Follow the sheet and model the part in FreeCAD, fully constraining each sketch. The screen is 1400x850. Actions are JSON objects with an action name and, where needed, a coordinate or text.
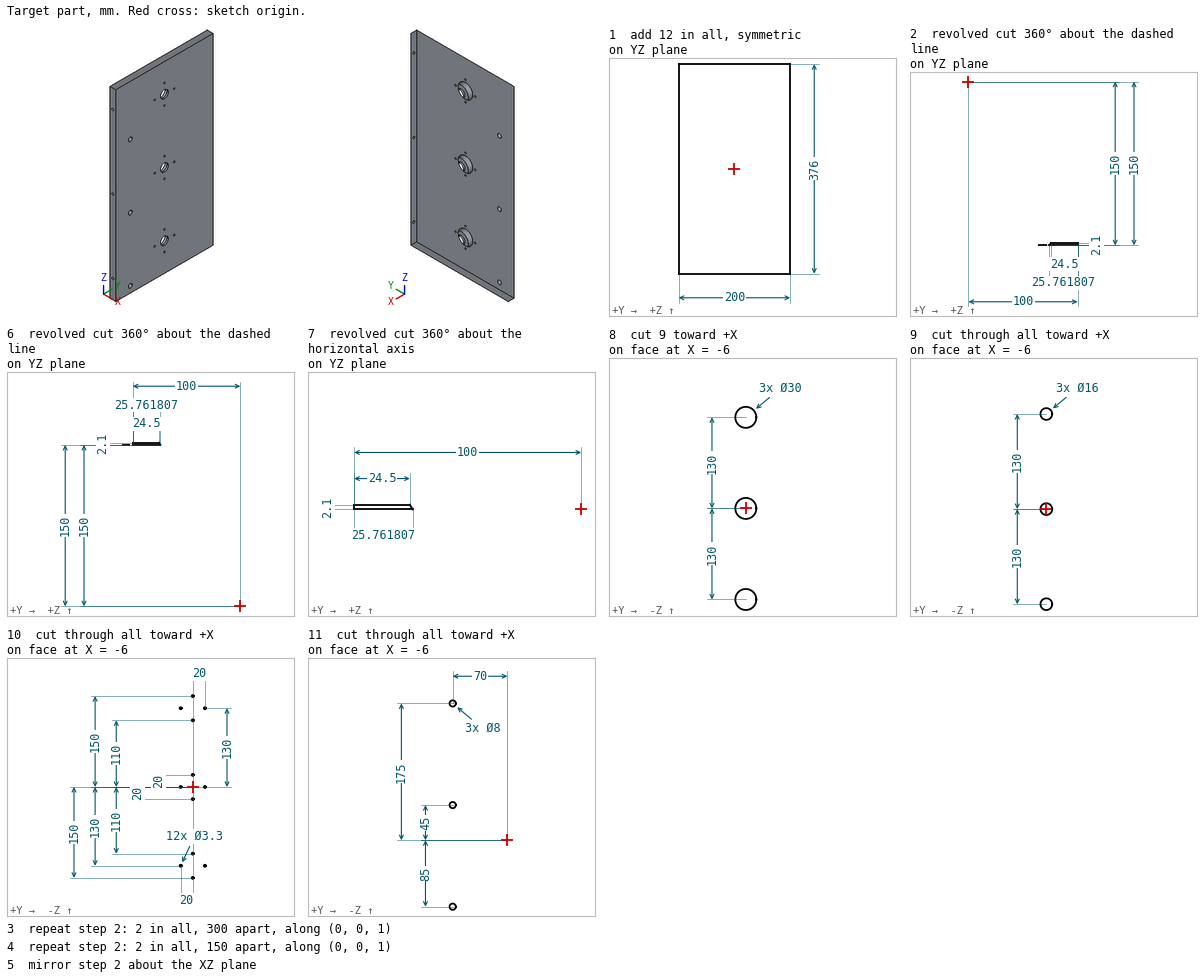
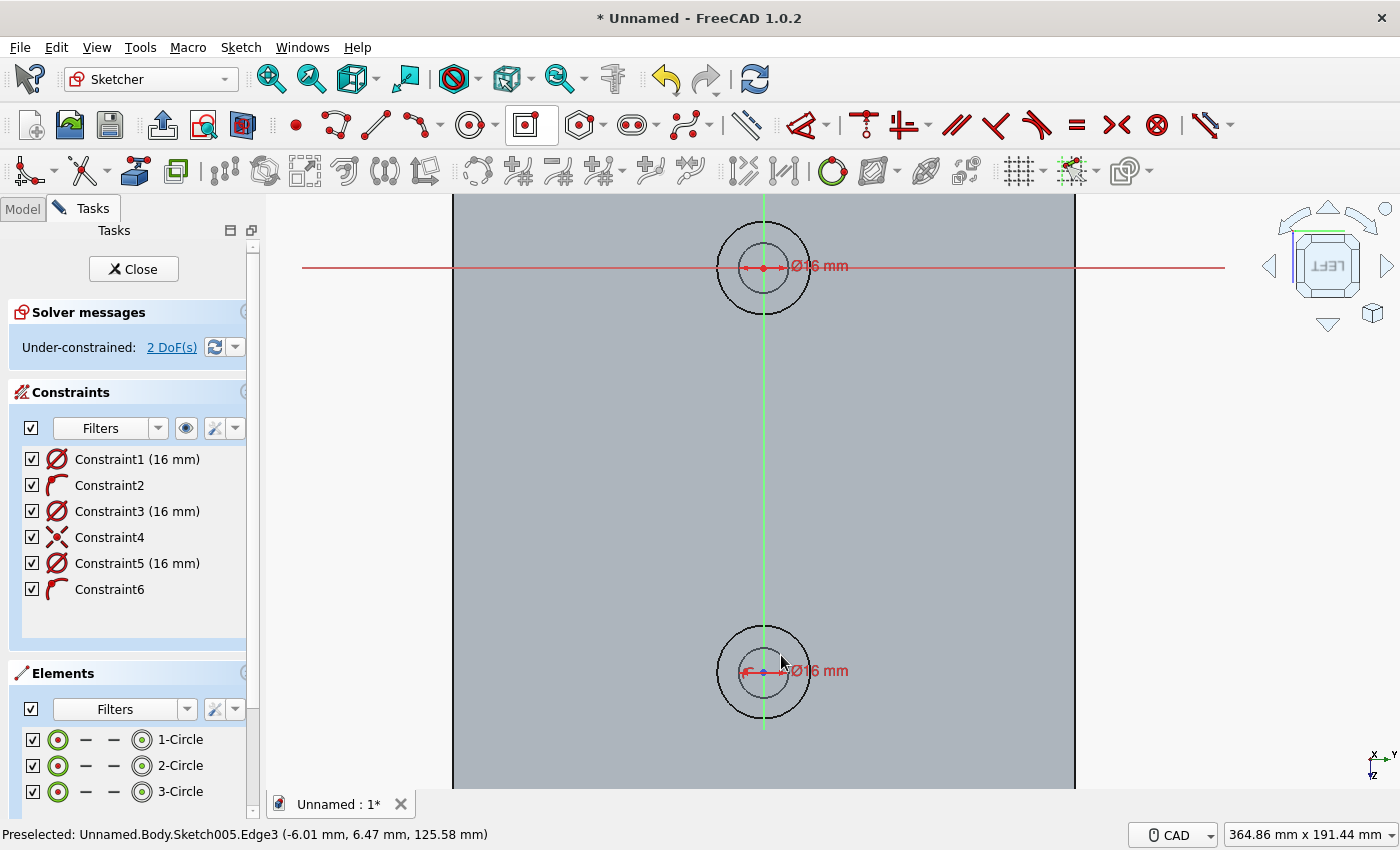
{"action": "left_click", "coordinate": [802, 126]}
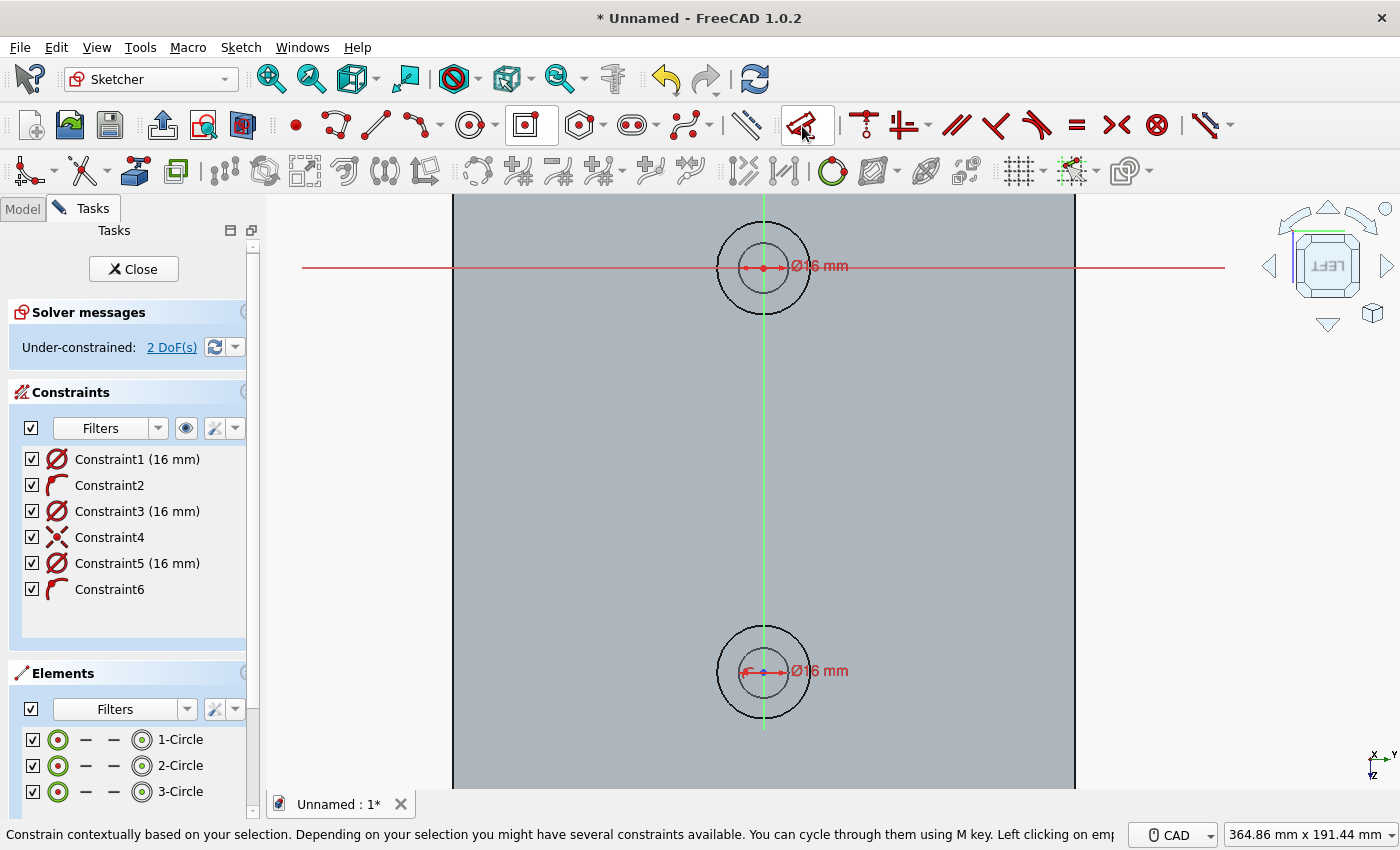
{"action": "scroll", "coordinate": [765, 674], "scroll_direction": "down", "scroll_amount": 4}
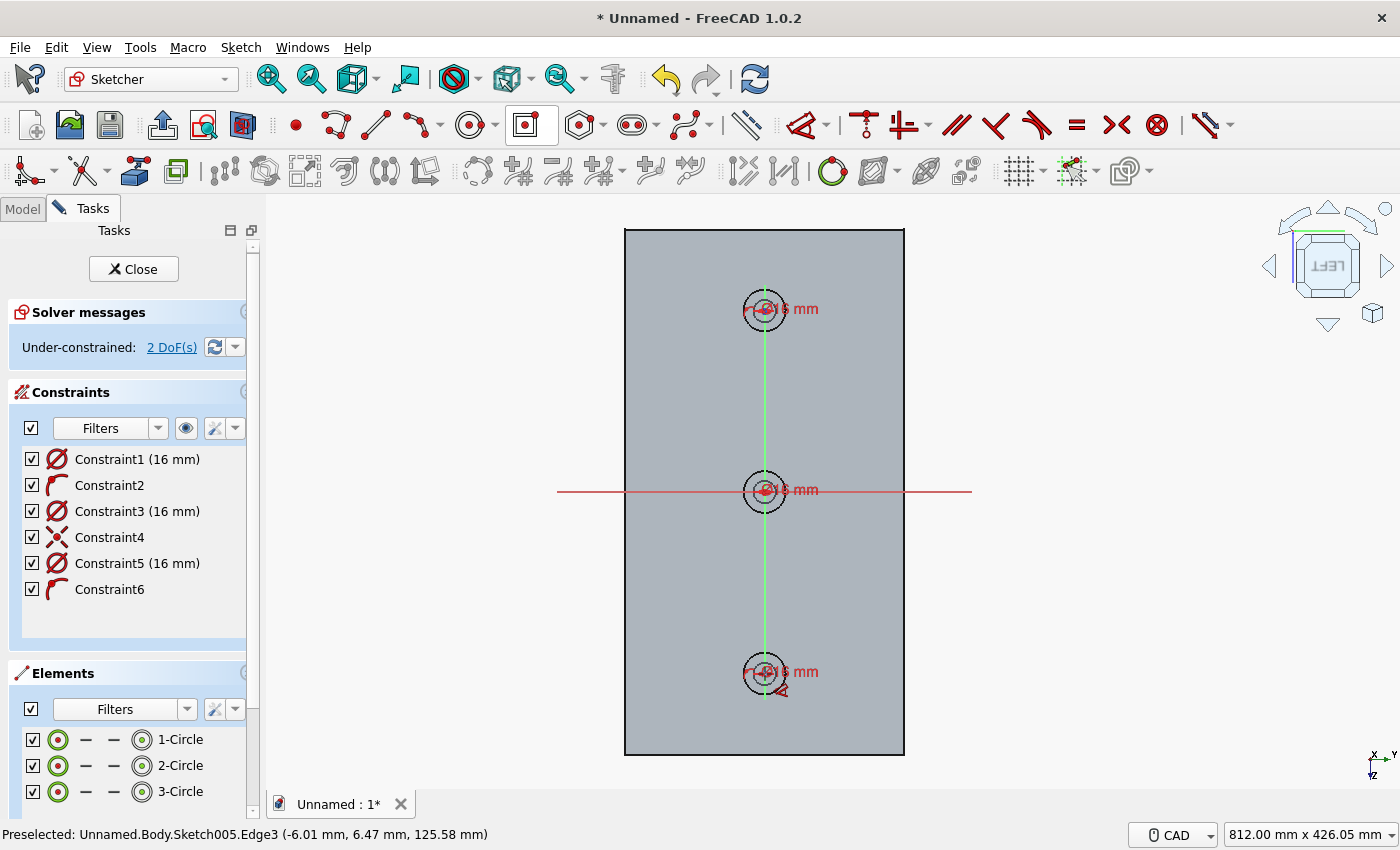
{"action": "left_click", "coordinate": [765, 311]}
{"action": "left_click", "coordinate": [799, 402]}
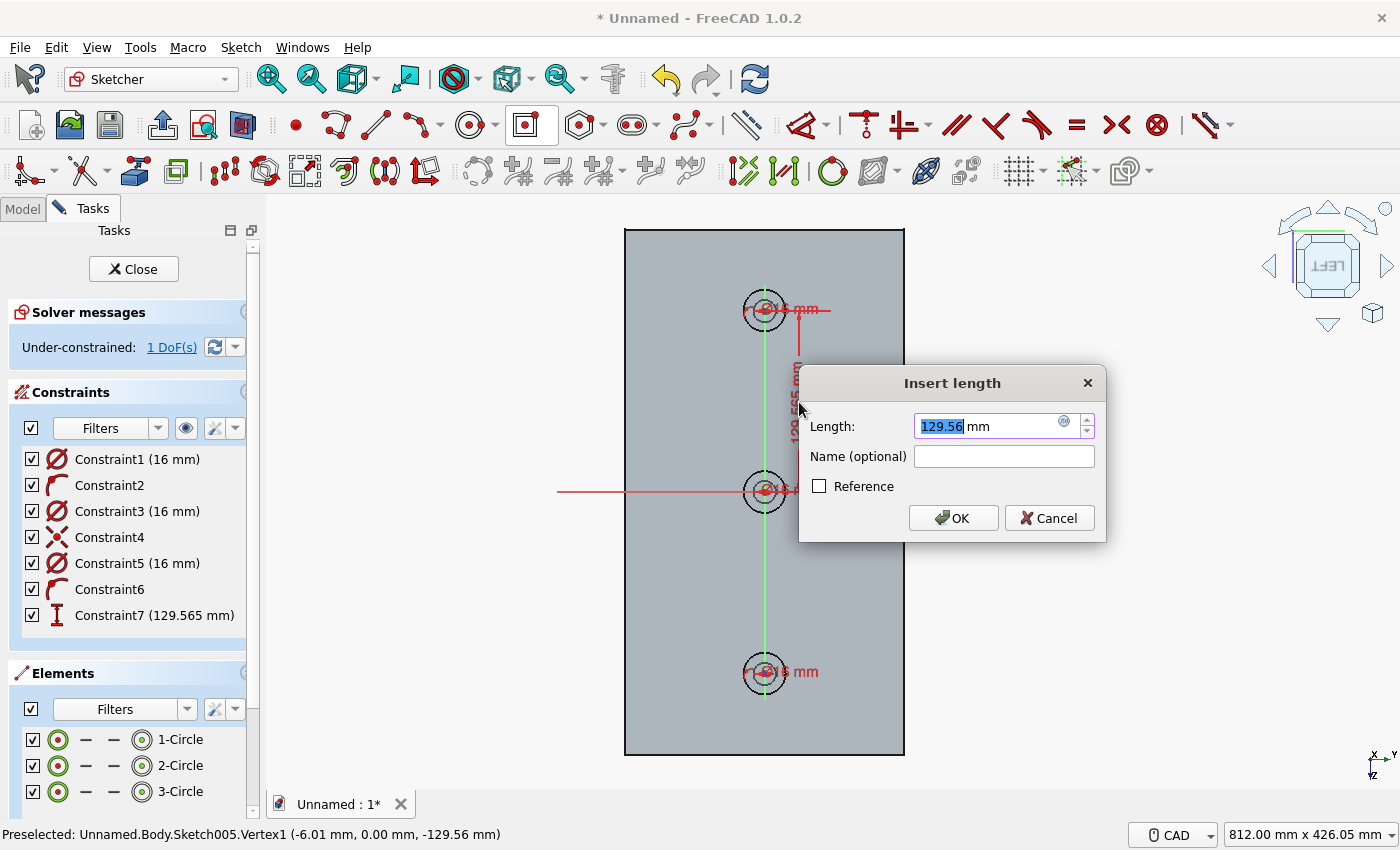
{"action": "type", "text": "130"}
{"action": "key", "text": "Return"}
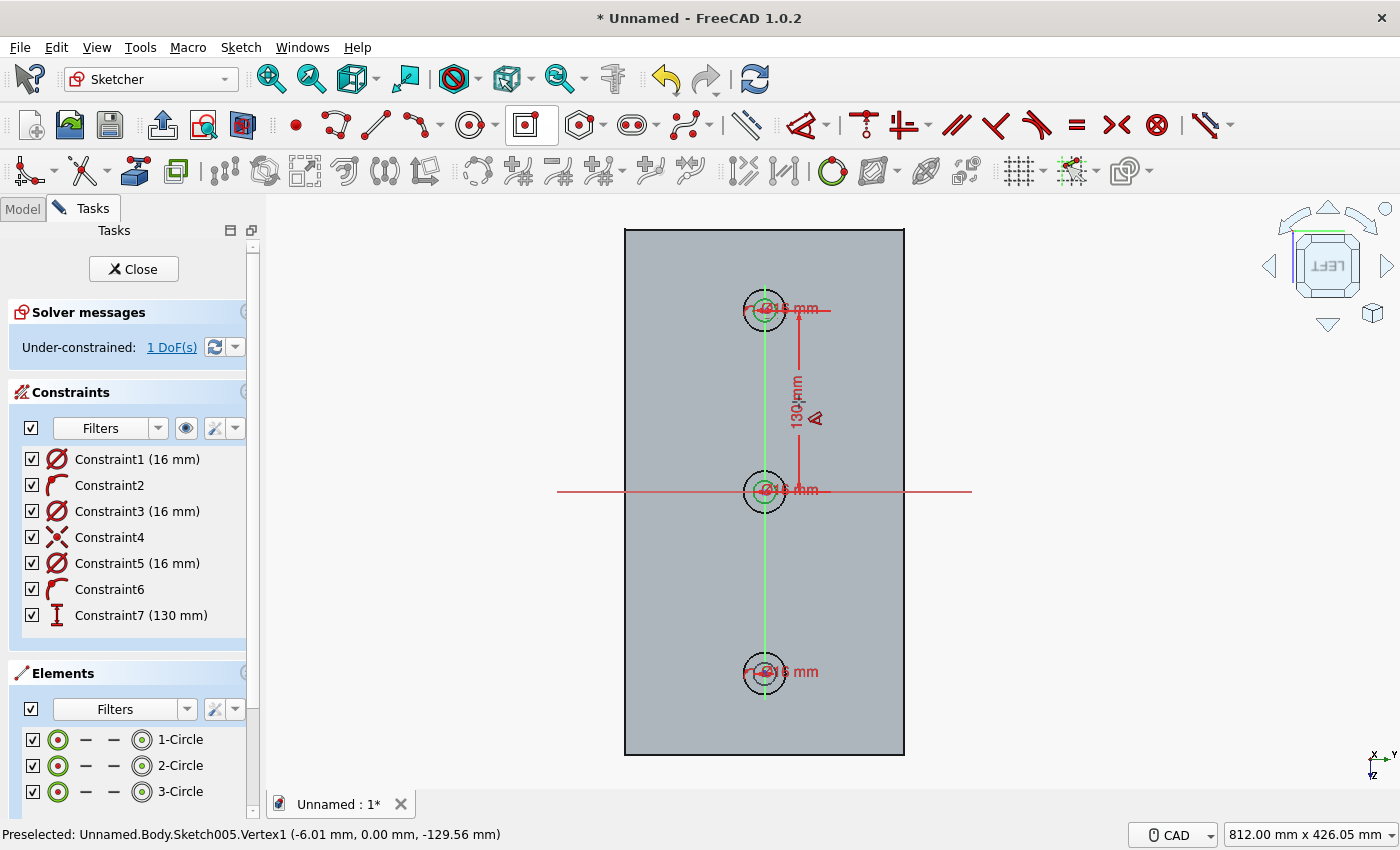
{"action": "left_click", "coordinate": [765, 674]}
{"action": "left_click", "coordinate": [799, 583]}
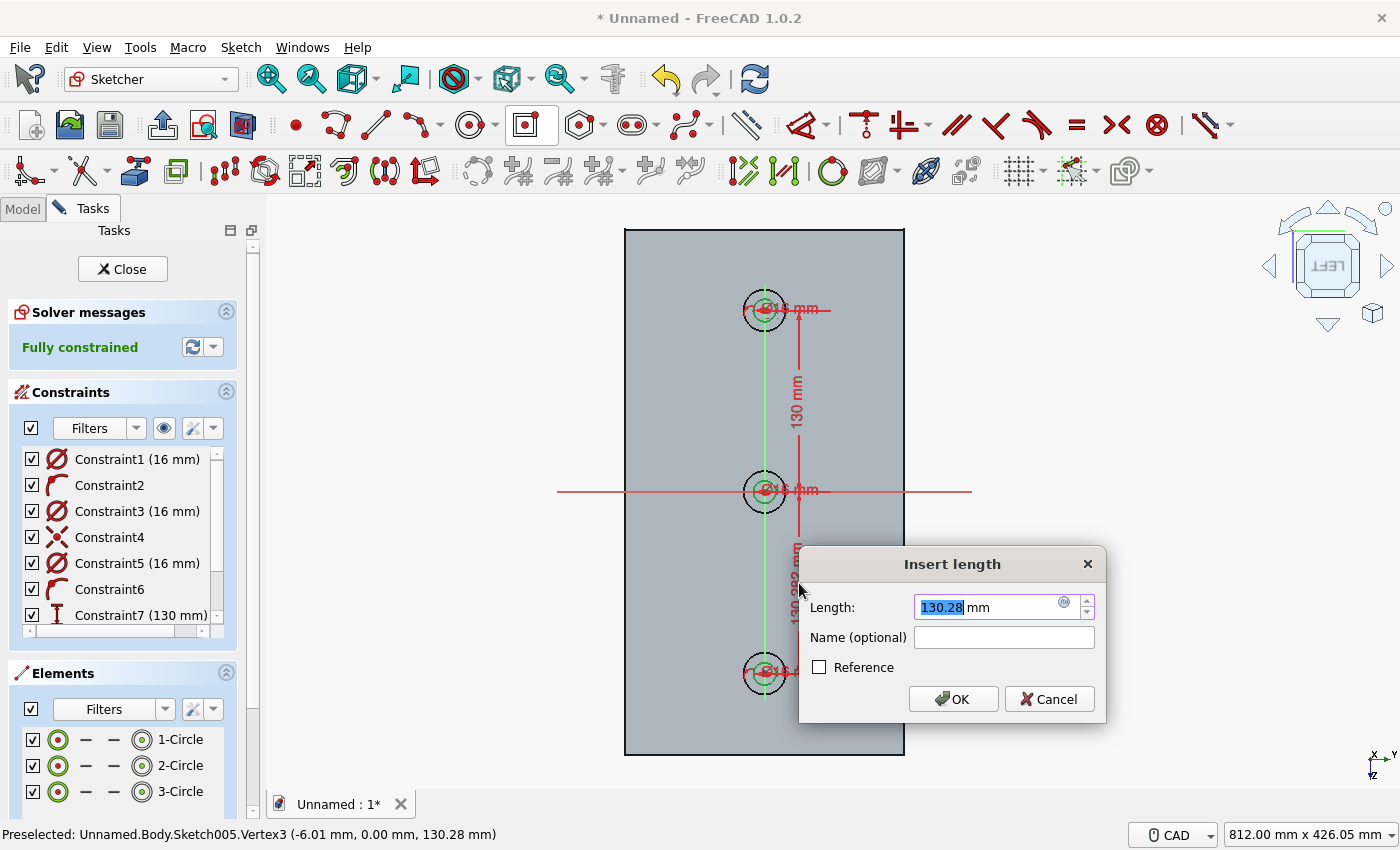
{"action": "type", "text": "130"}
{"action": "key", "text": "Return"}
{"action": "key", "text": "Escape"}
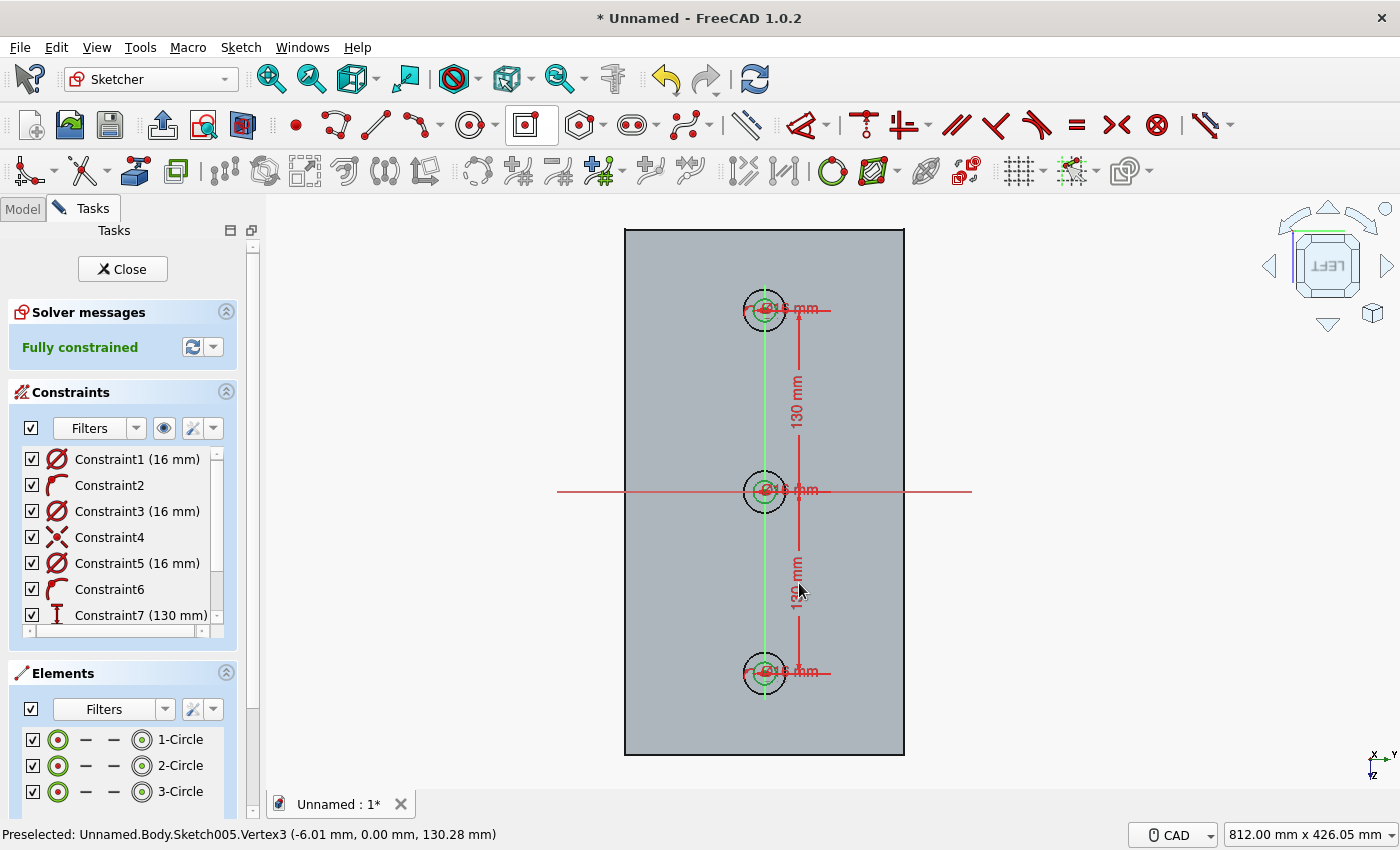
{"action": "left_click", "coordinate": [123, 269]}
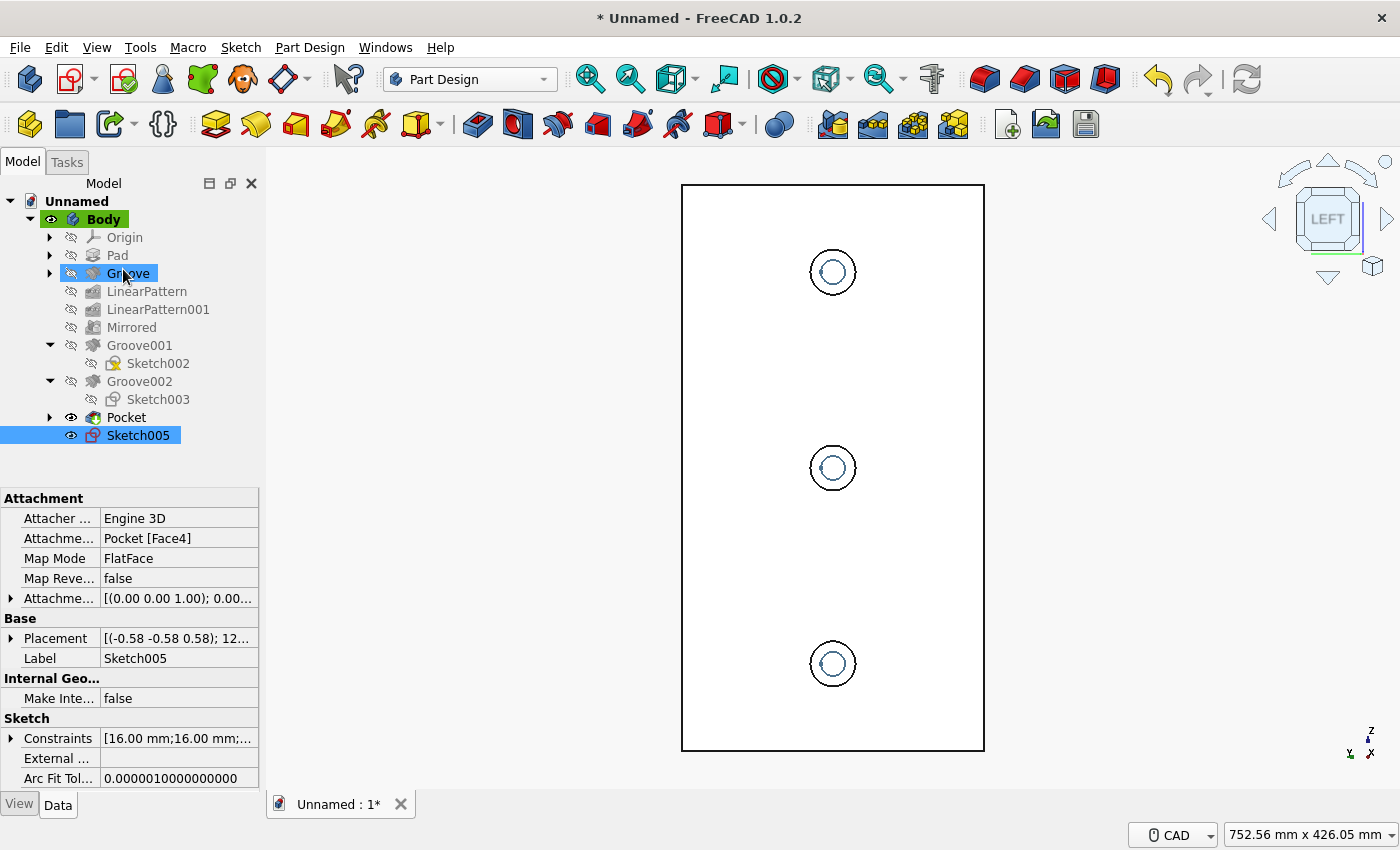
{"action": "left_click", "coordinate": [478, 124]}